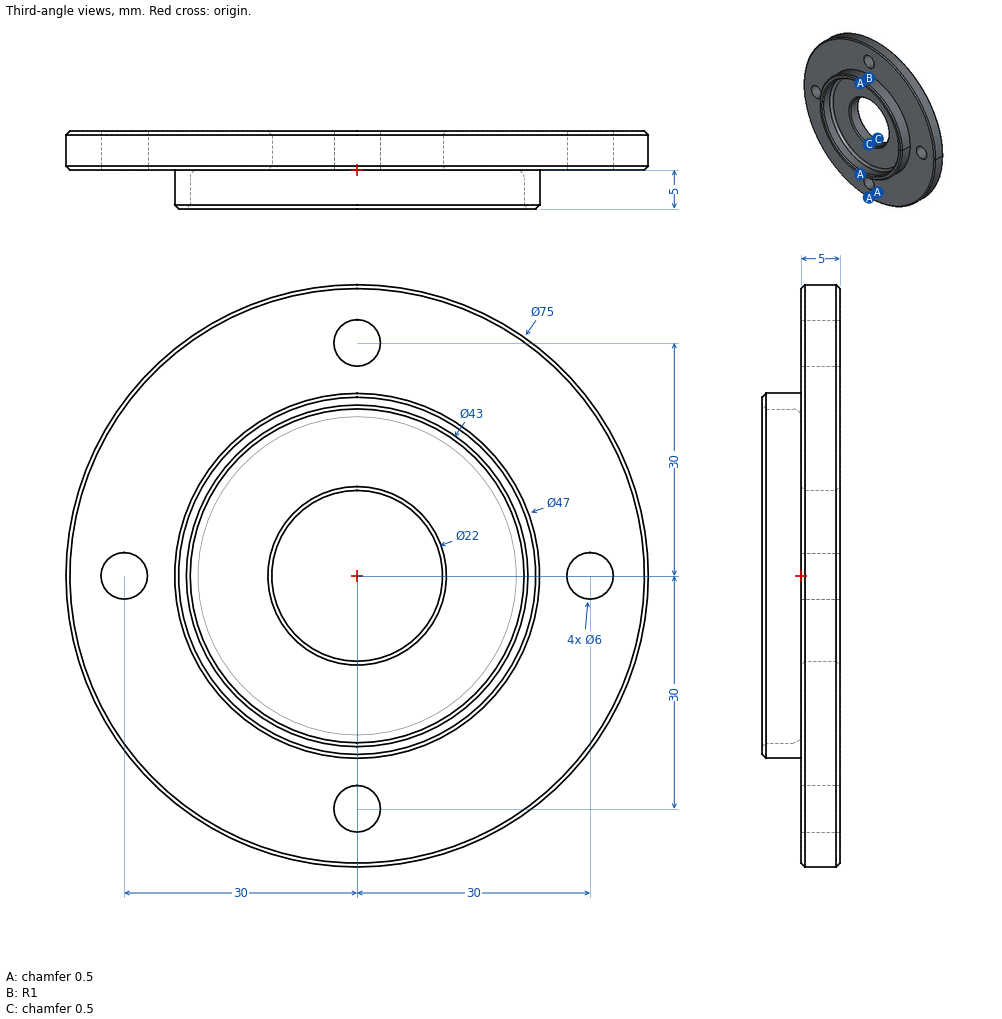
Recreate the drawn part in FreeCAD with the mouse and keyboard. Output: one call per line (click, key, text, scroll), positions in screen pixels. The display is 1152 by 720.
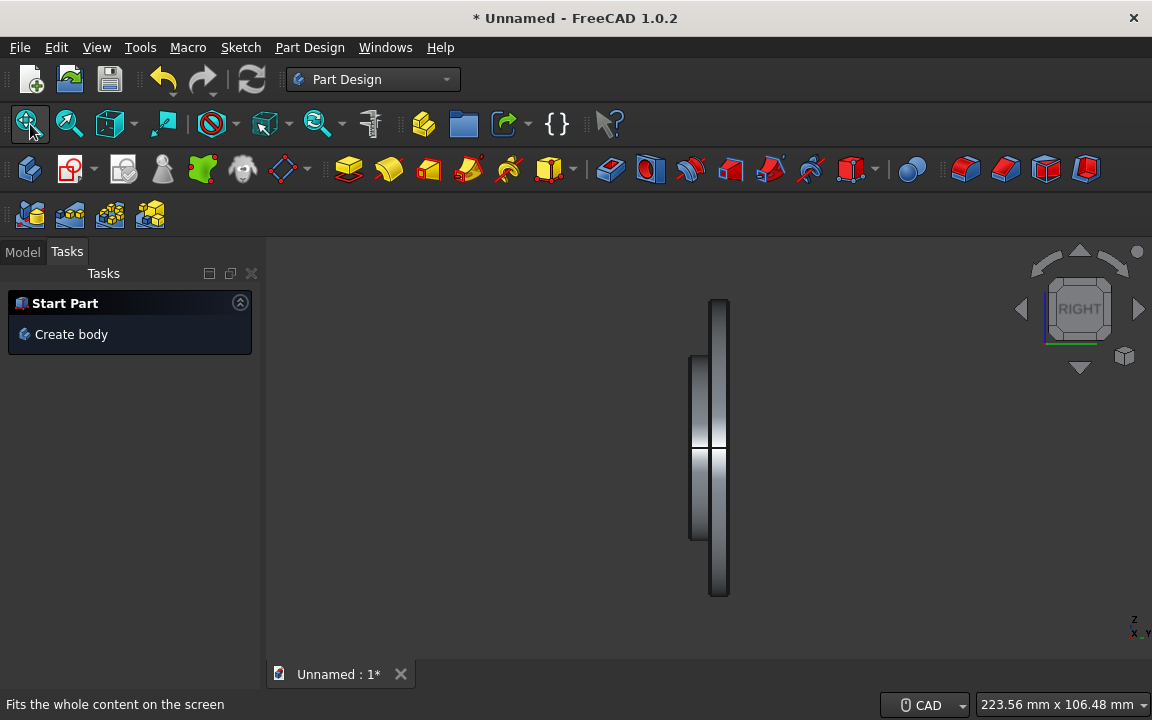
key(5)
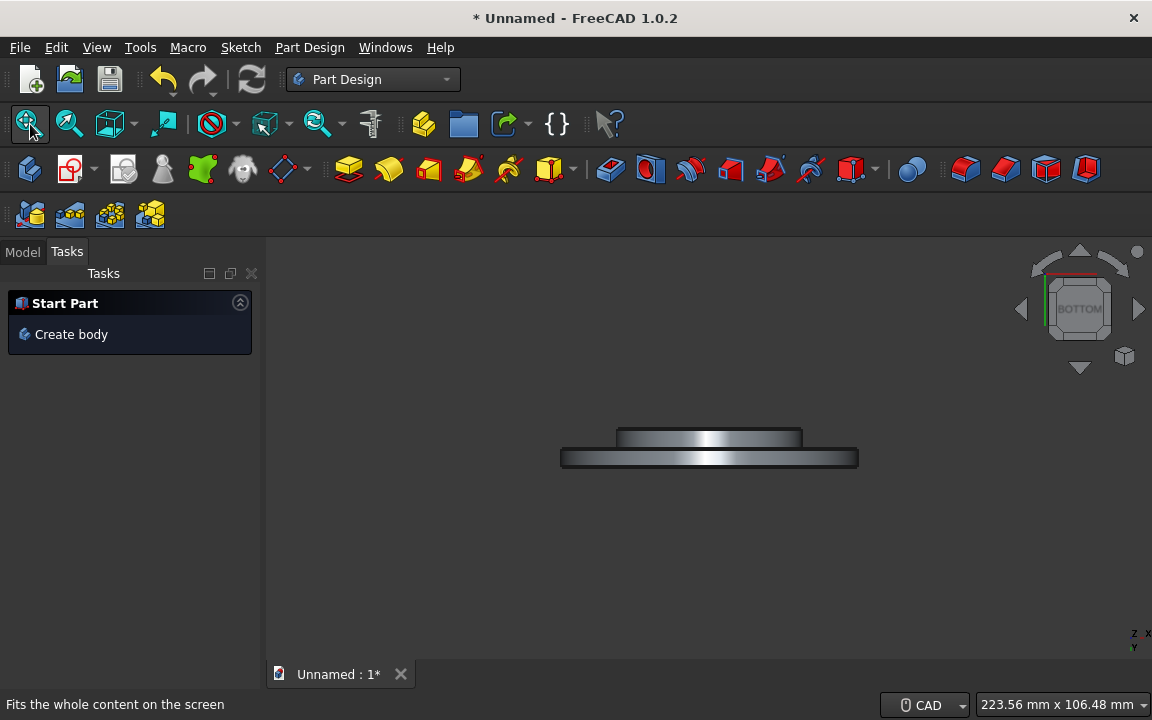
click(30, 124)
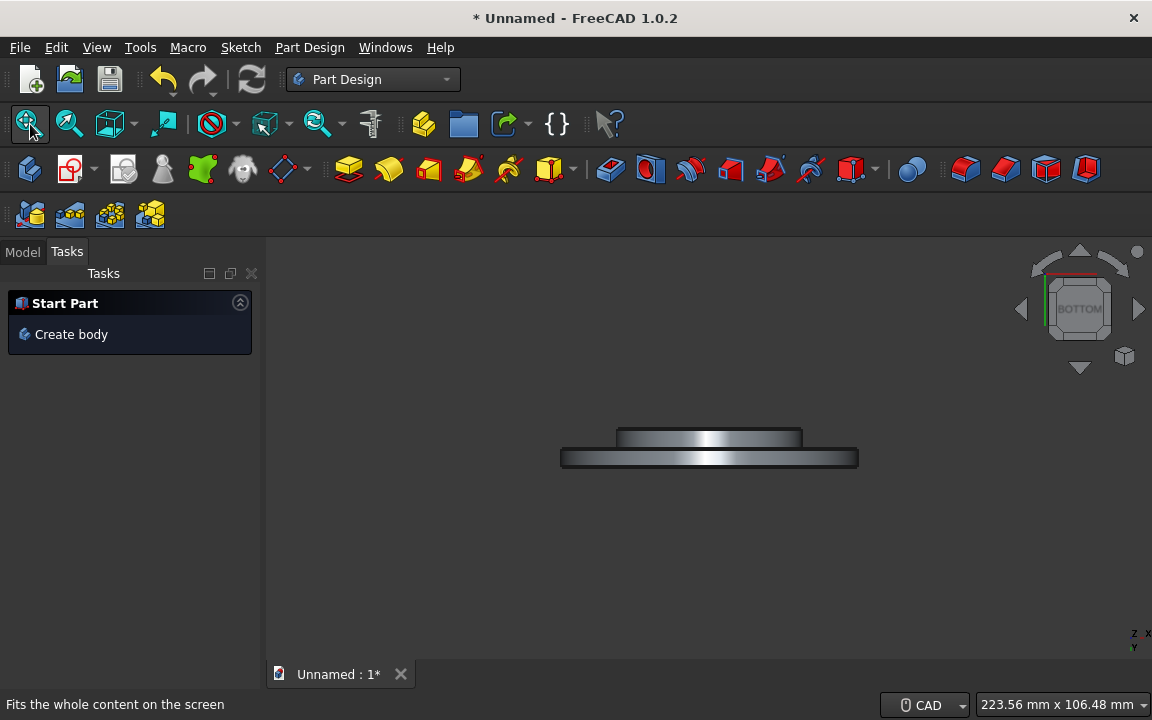
key(4)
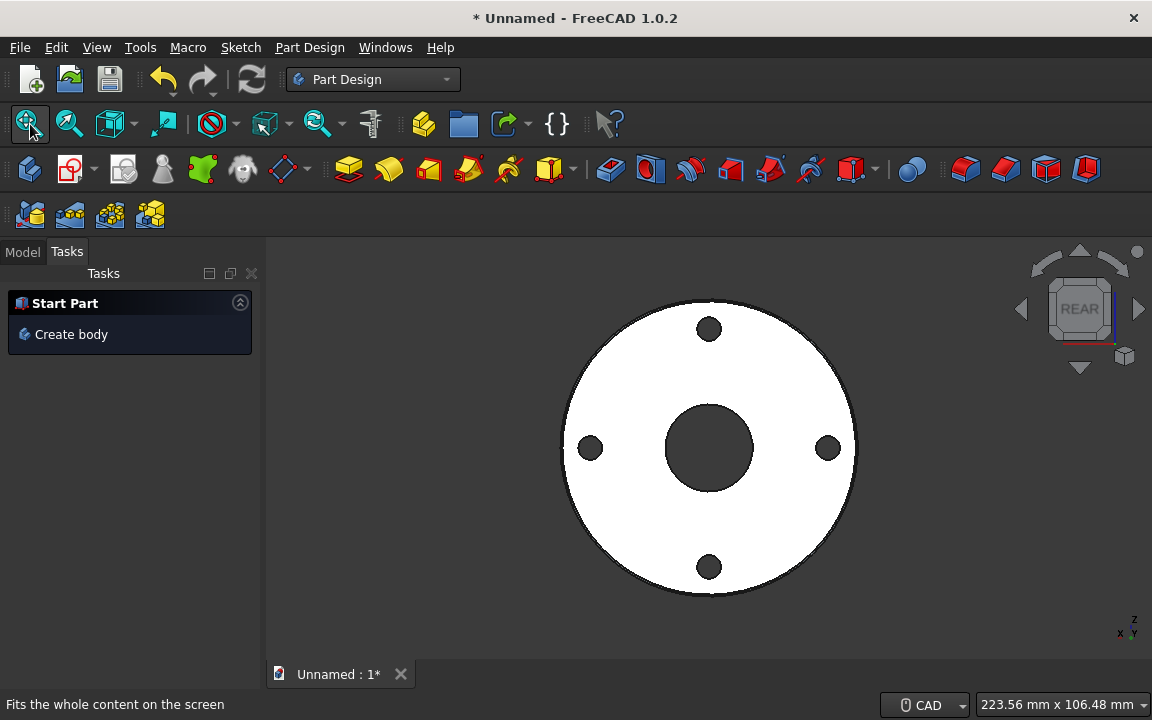
key(6)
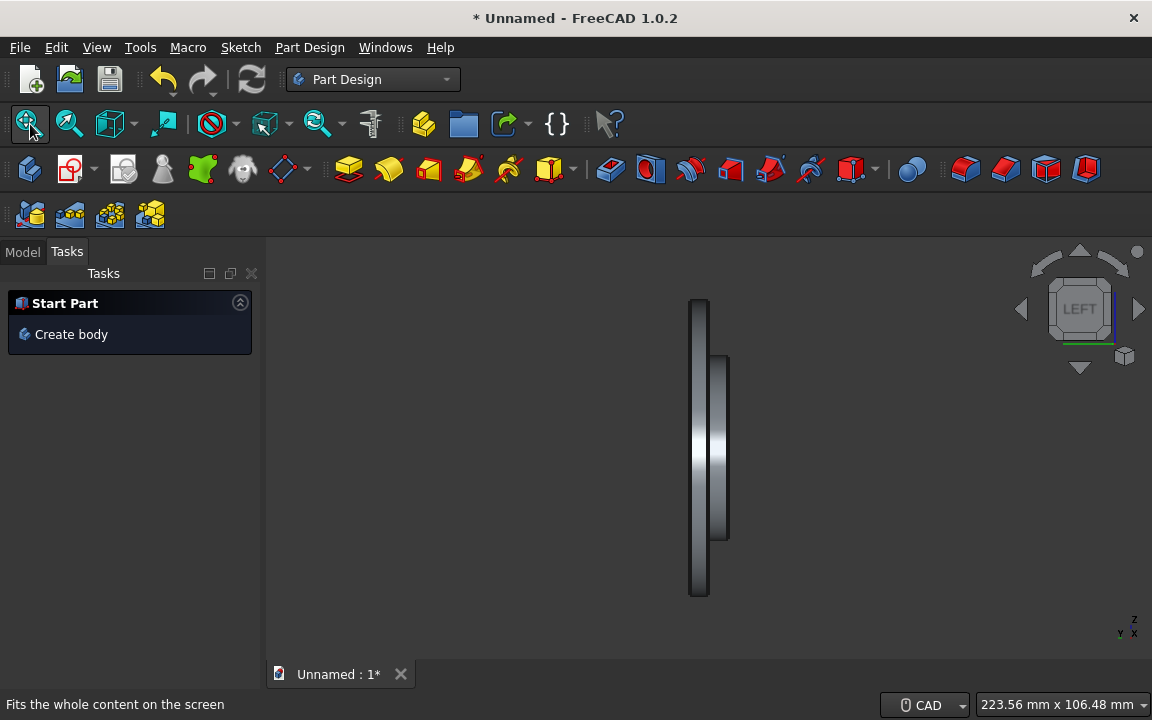
key(v)
key(3)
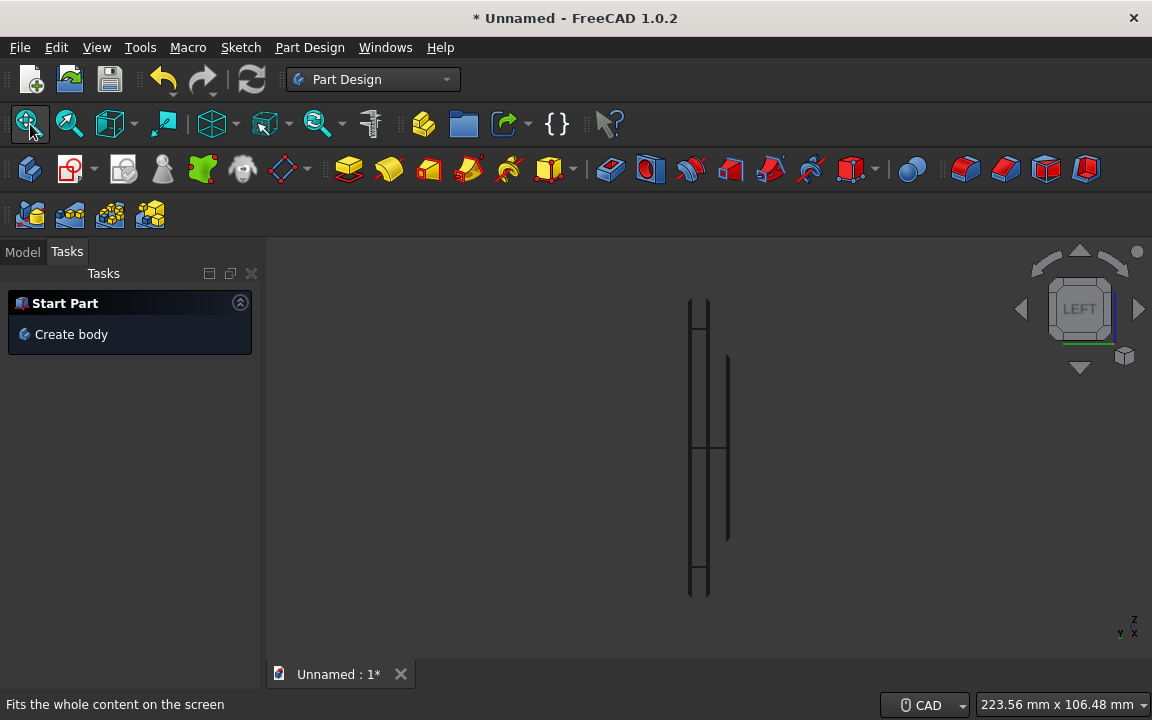
key(0)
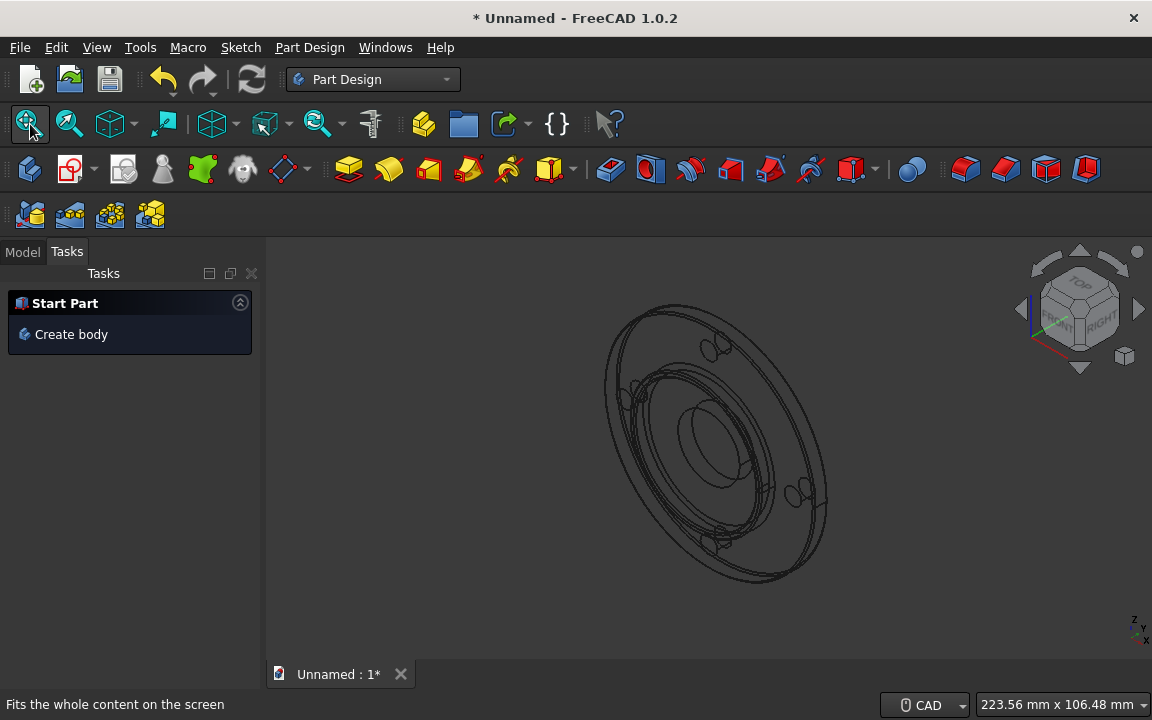
click(649, 412)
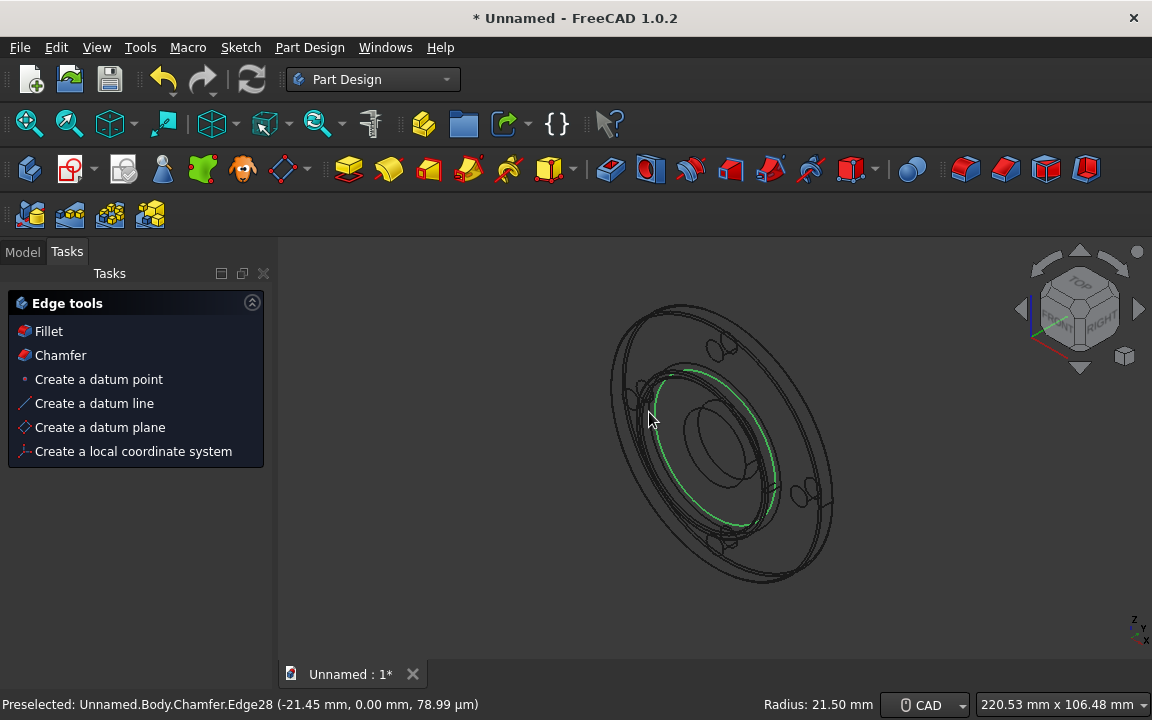
key(v)
key(1)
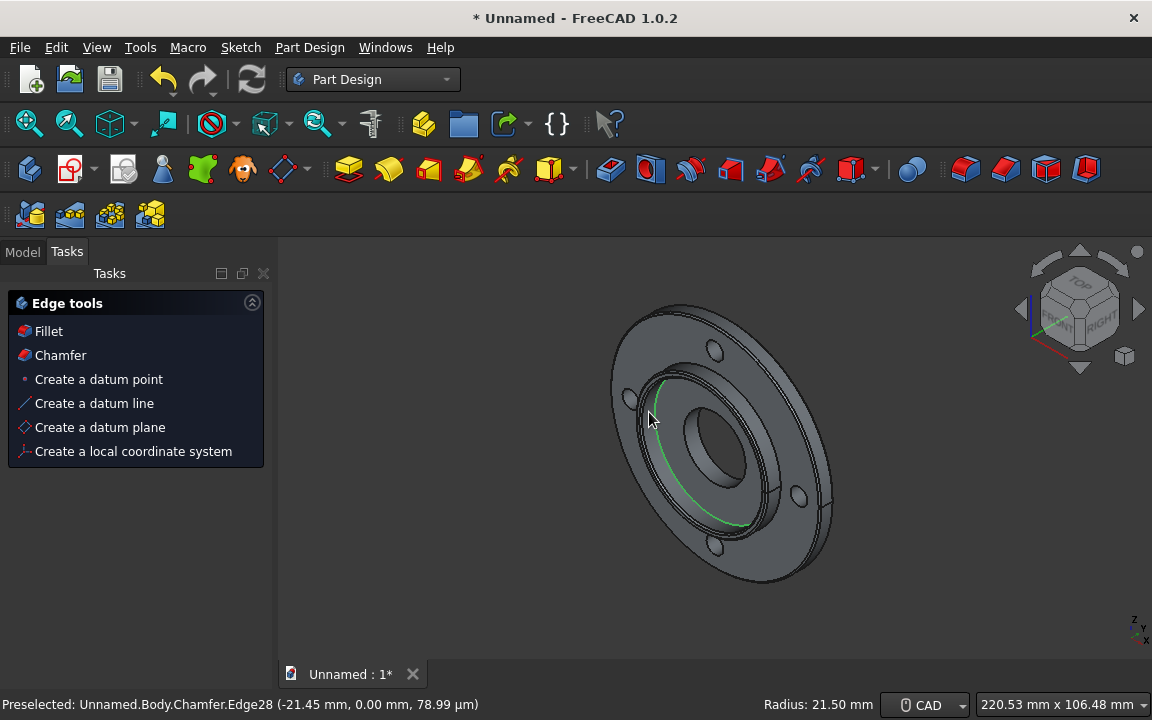
click(966, 170)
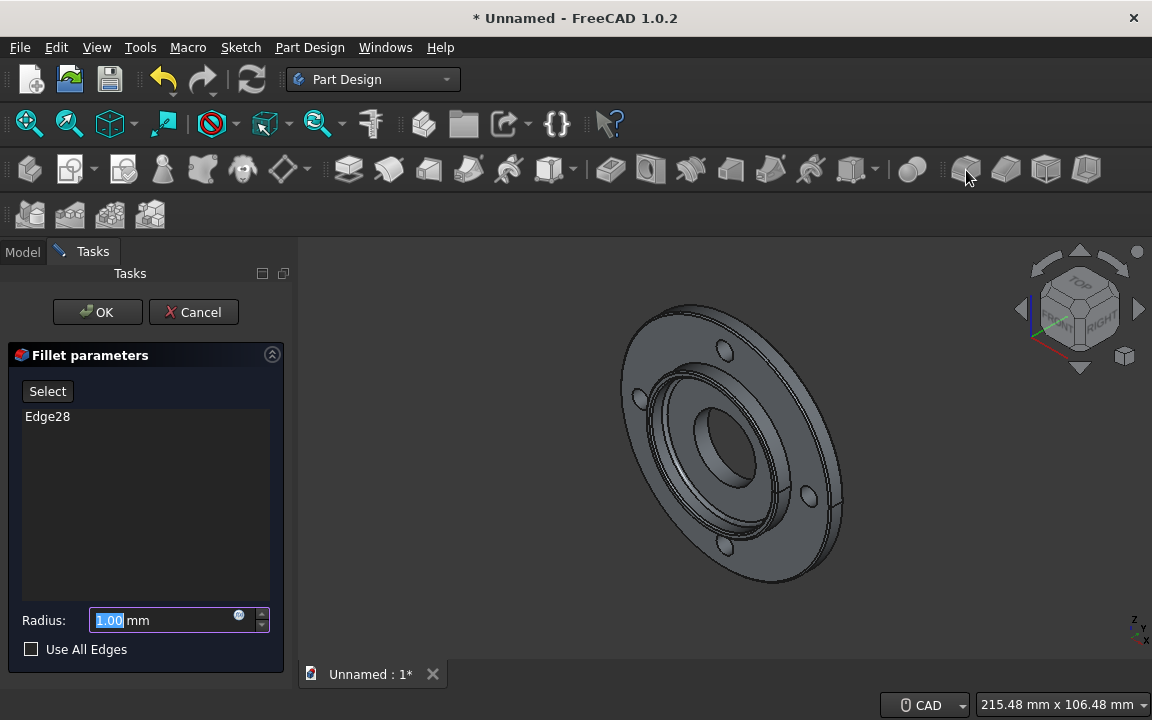
text(1)
key(Tab)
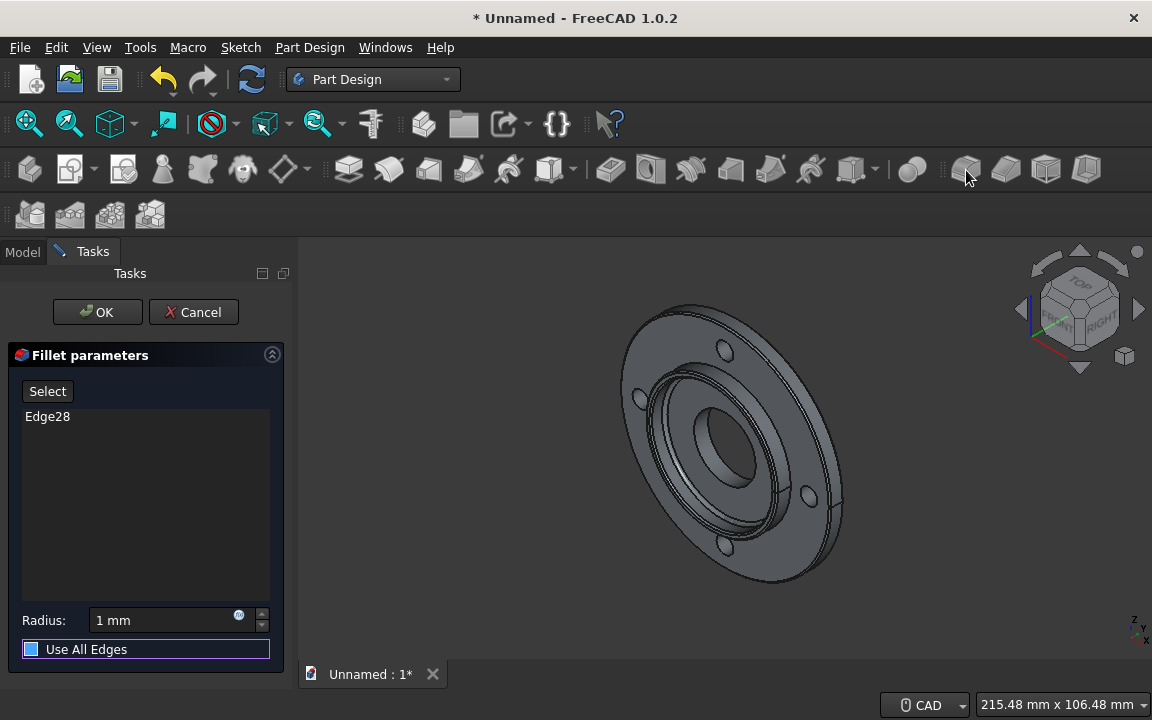
click(98, 312)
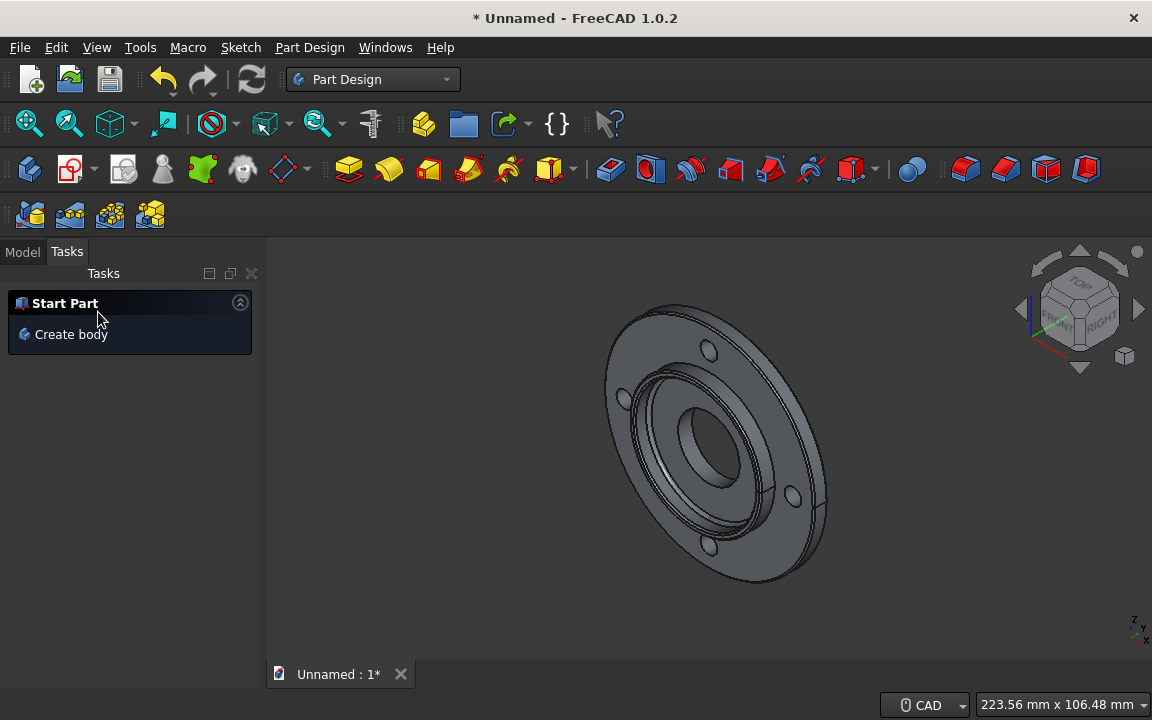
click(678, 429)